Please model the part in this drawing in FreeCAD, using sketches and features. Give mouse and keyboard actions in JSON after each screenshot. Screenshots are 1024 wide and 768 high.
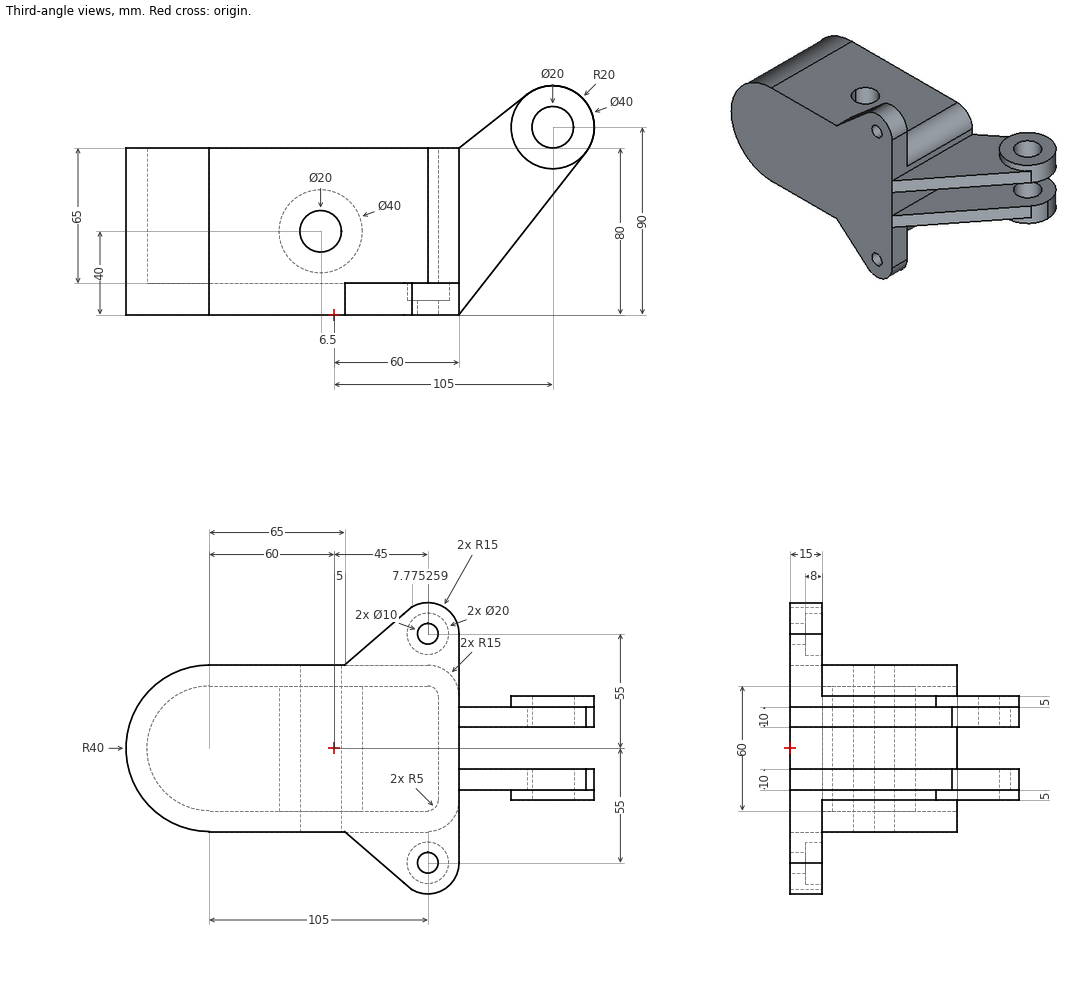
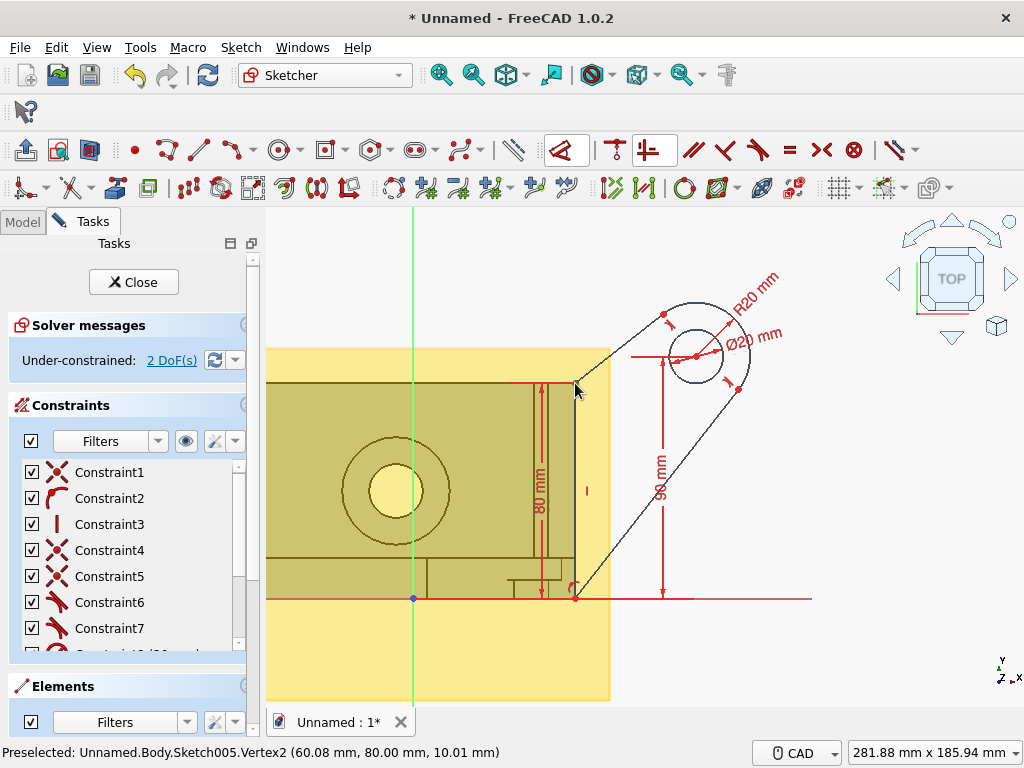
{"action": "key", "text": "l"}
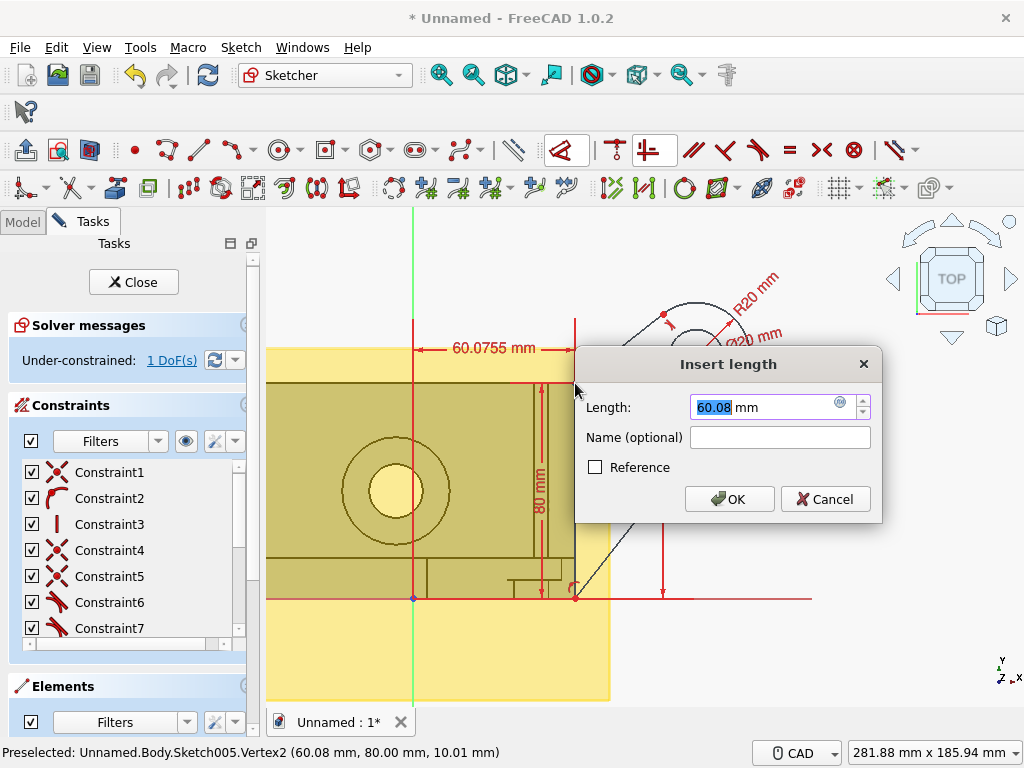
{"action": "type", "text": "60"}
{"action": "key", "text": "Return"}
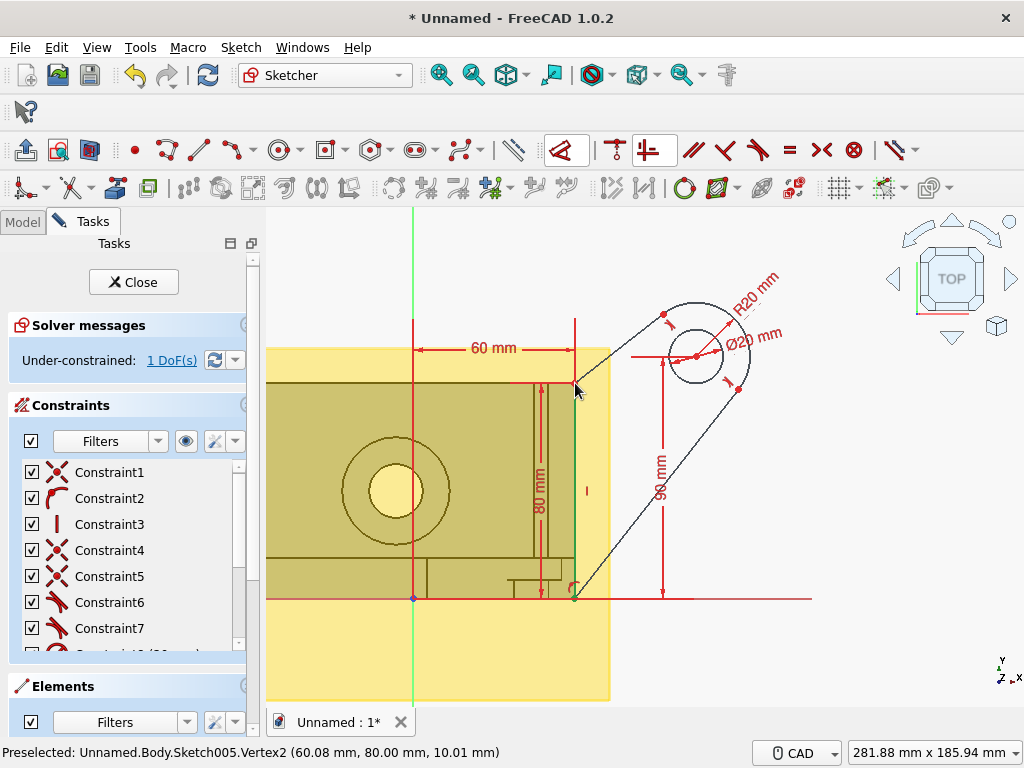
{"action": "left_click", "coordinate": [696, 357]}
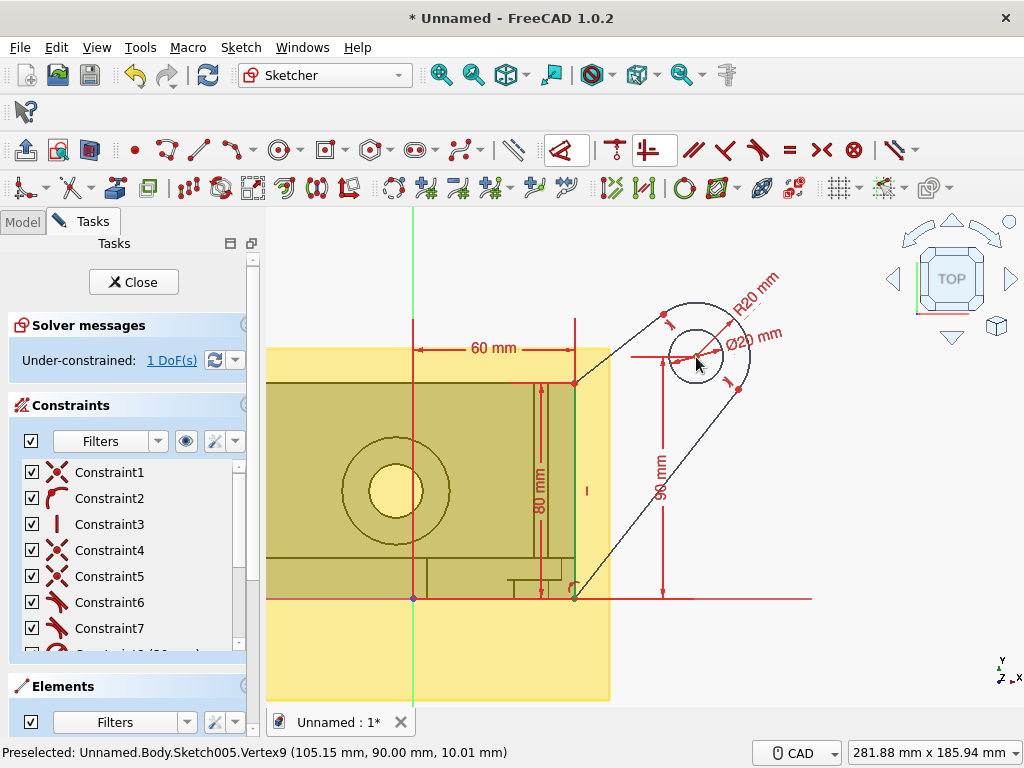
{"action": "left_click", "coordinate": [584, 150]}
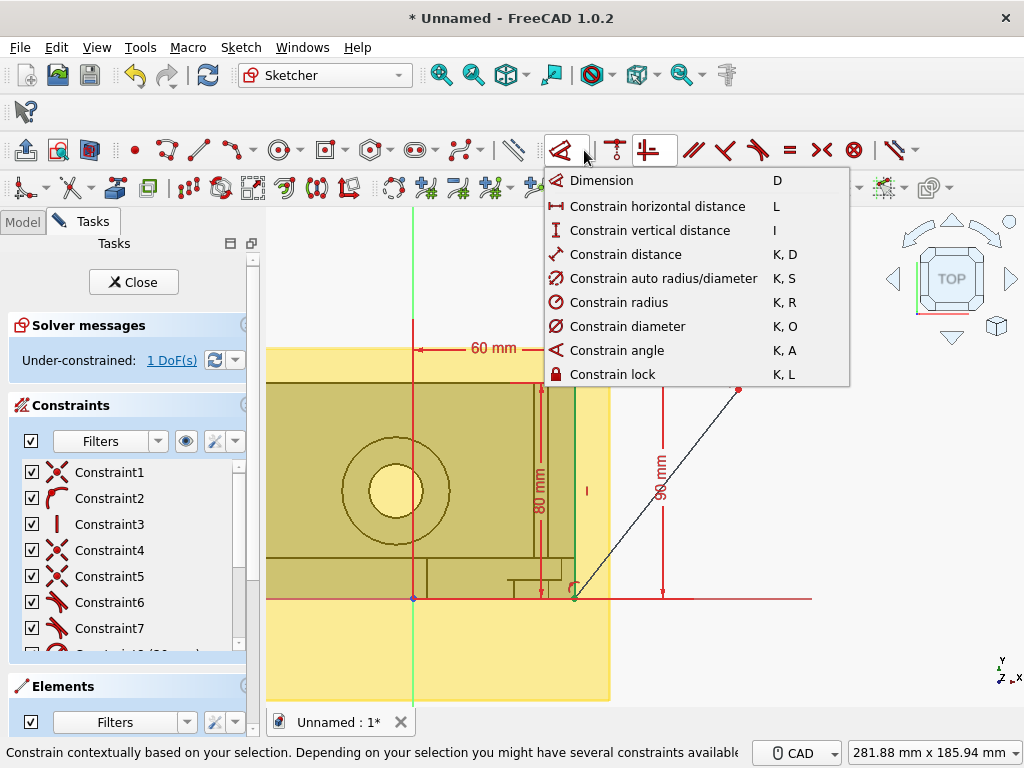
{"action": "left_click", "coordinate": [697, 206]}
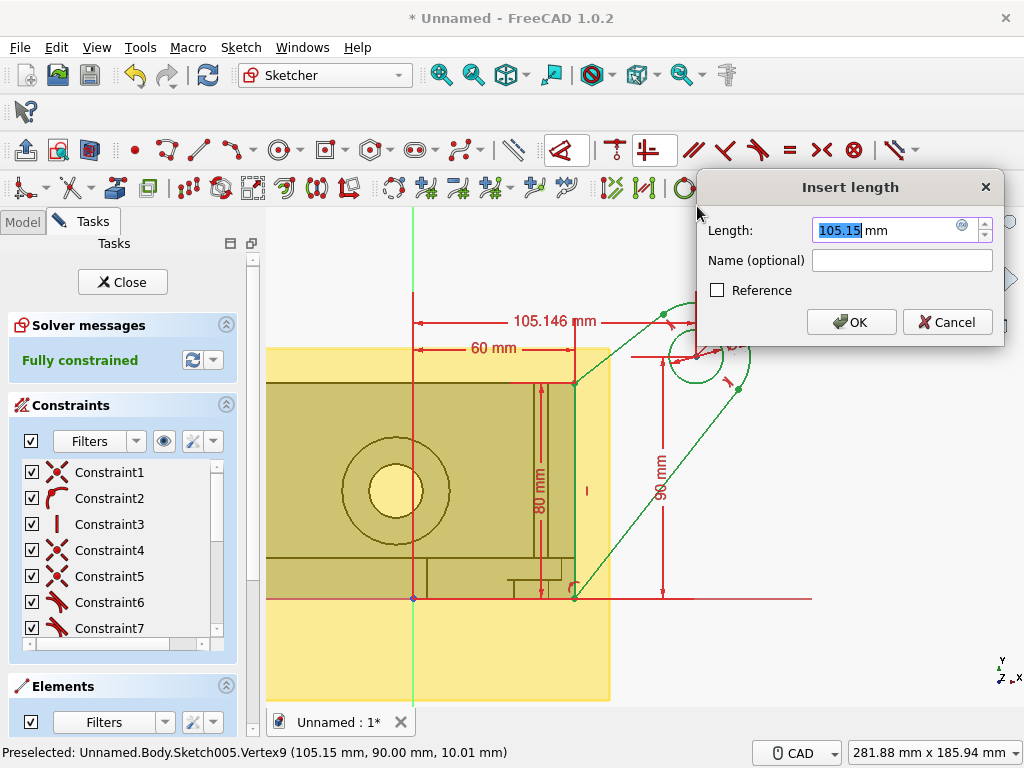
{"action": "type", "text": "105"}
{"action": "key", "text": "Return"}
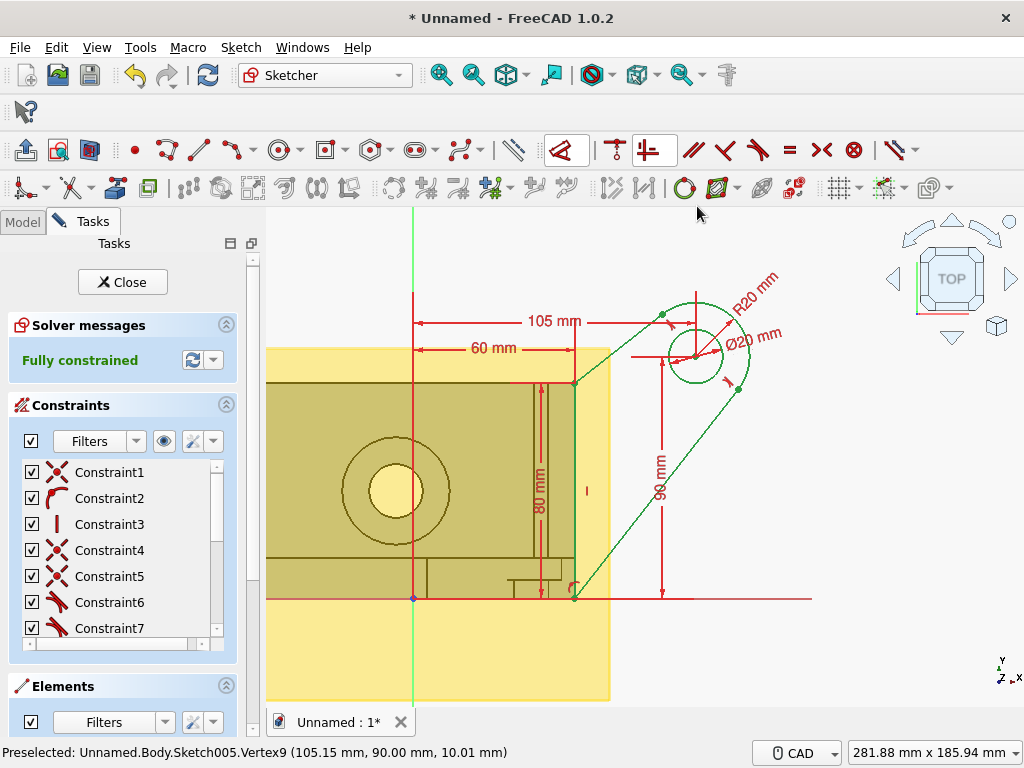
{"action": "left_click", "coordinate": [123, 282]}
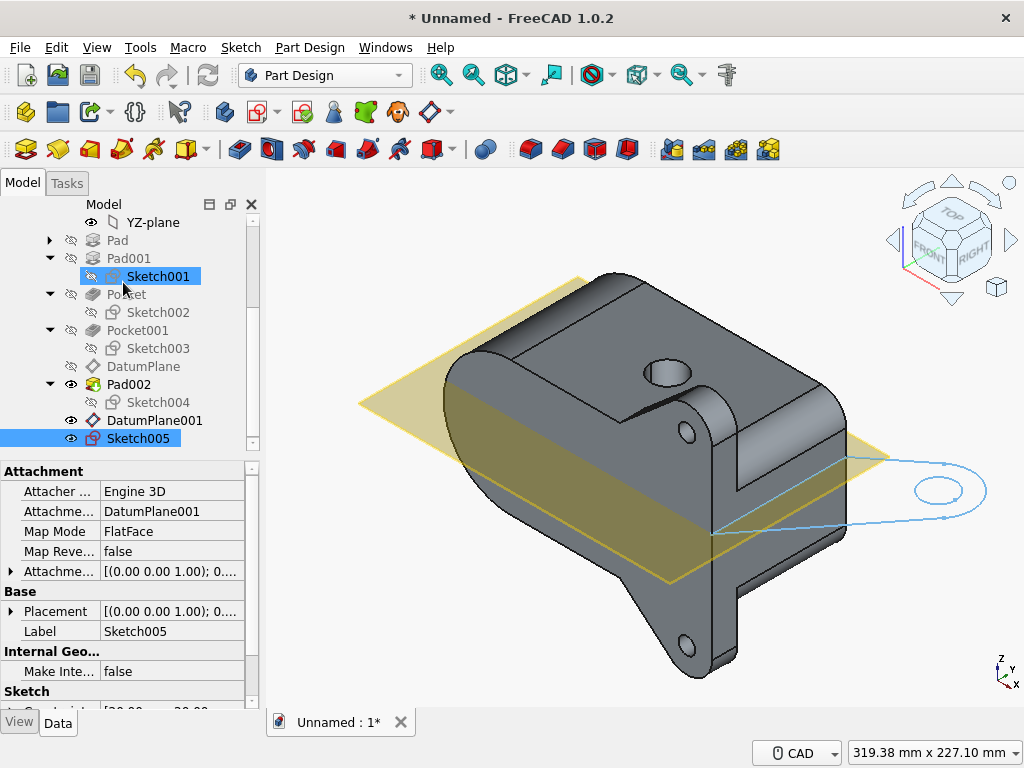
{"action": "left_click", "coordinate": [26, 150]}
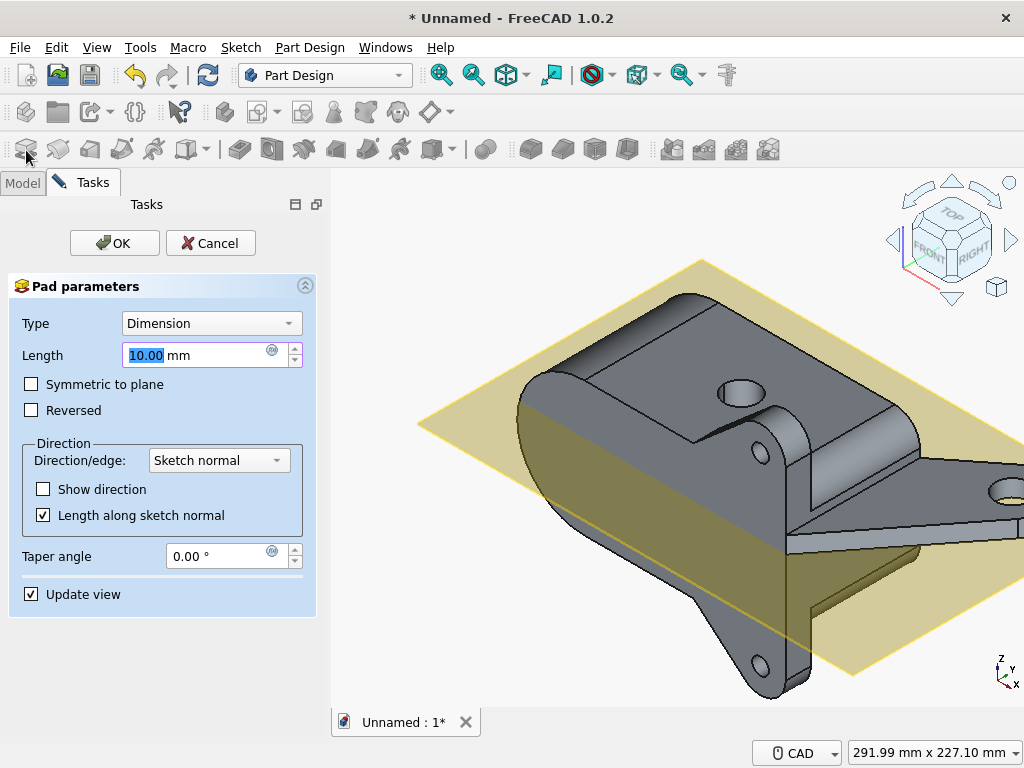
{"action": "type", "text": "10"}
{"action": "key", "text": "Tab"}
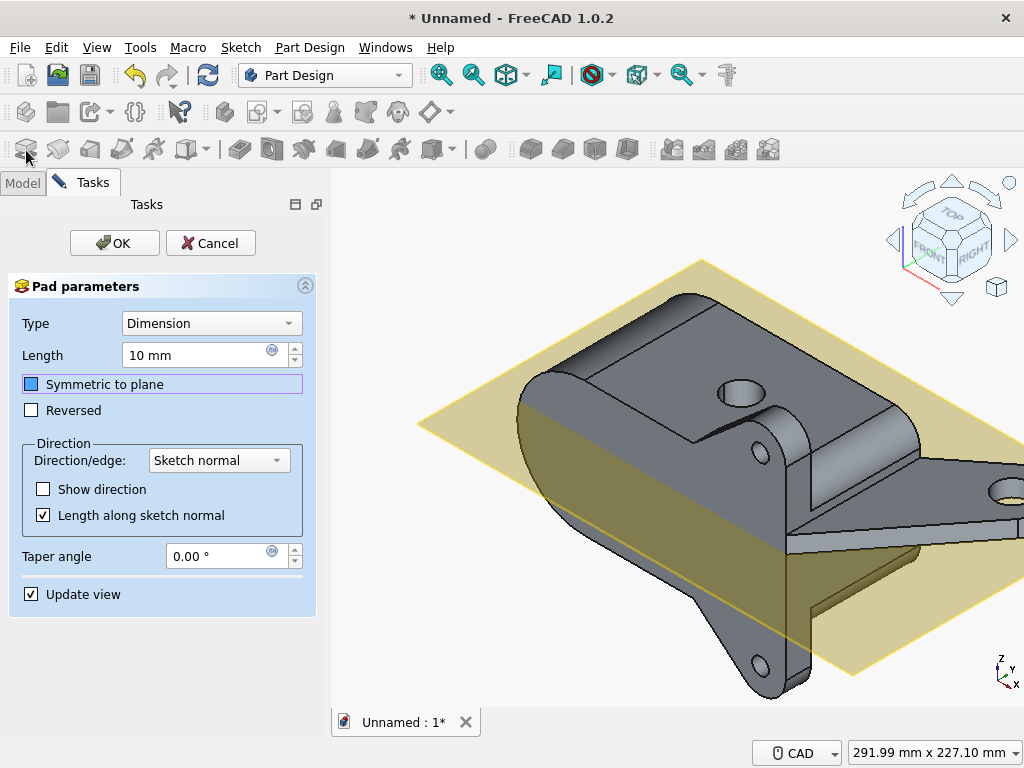
{"action": "left_click", "coordinate": [115, 243]}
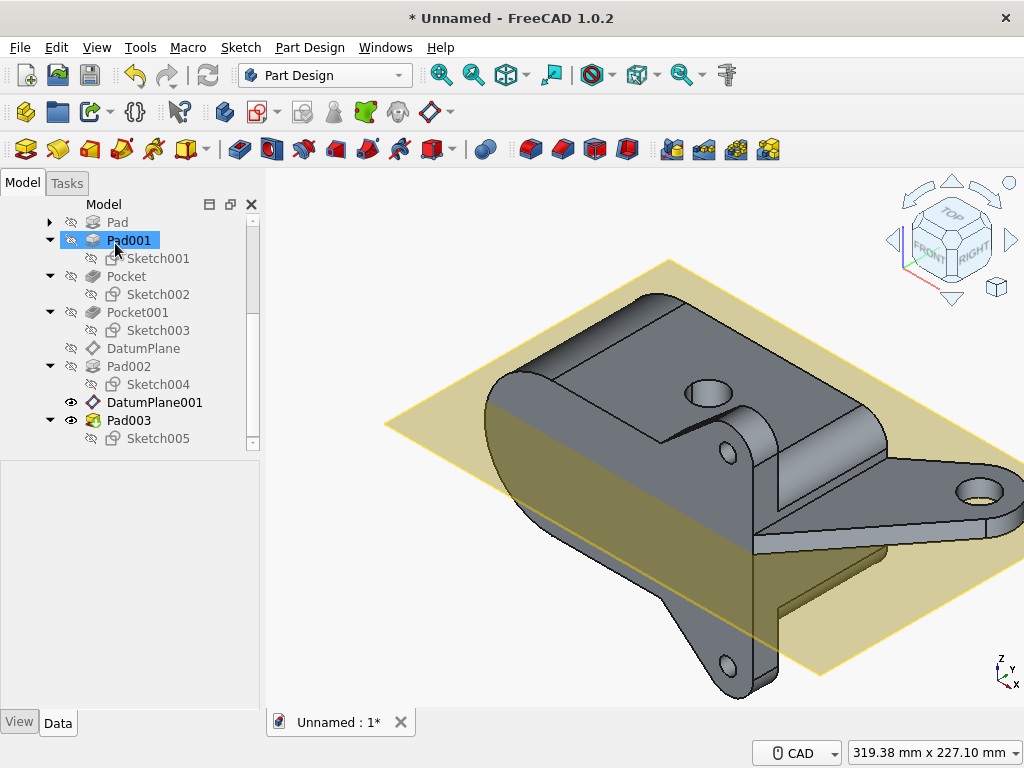
{"action": "left_click", "coordinate": [116, 402]}
{"action": "key", "text": "space"}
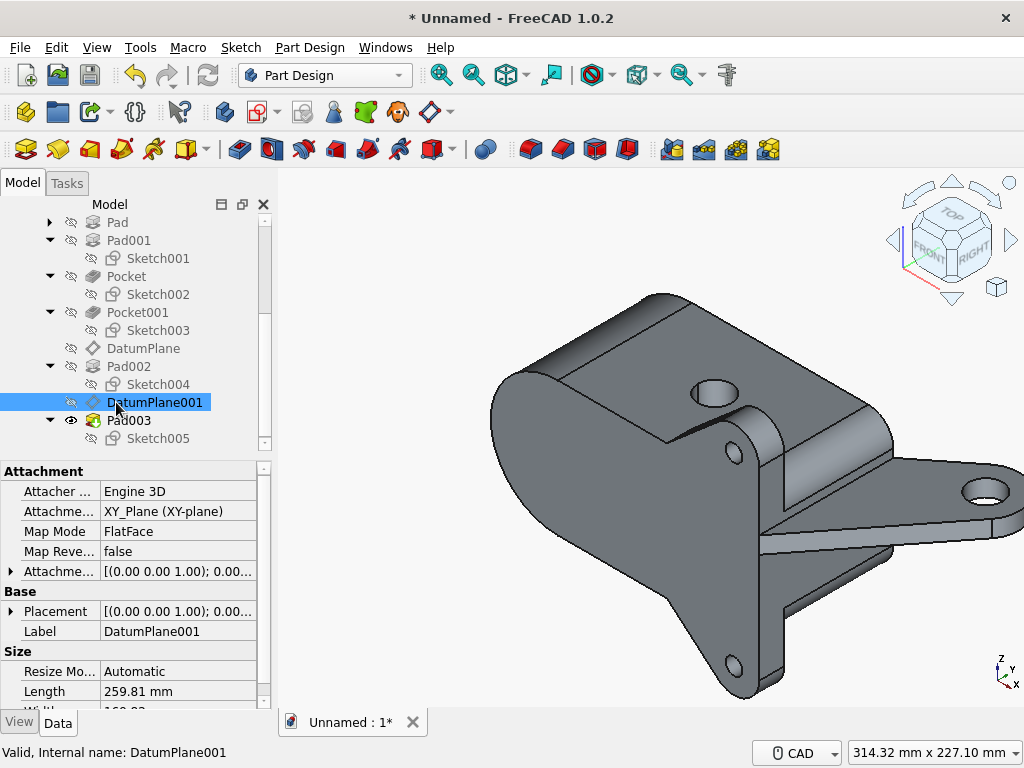
{"action": "left_click", "coordinate": [442, 76]}